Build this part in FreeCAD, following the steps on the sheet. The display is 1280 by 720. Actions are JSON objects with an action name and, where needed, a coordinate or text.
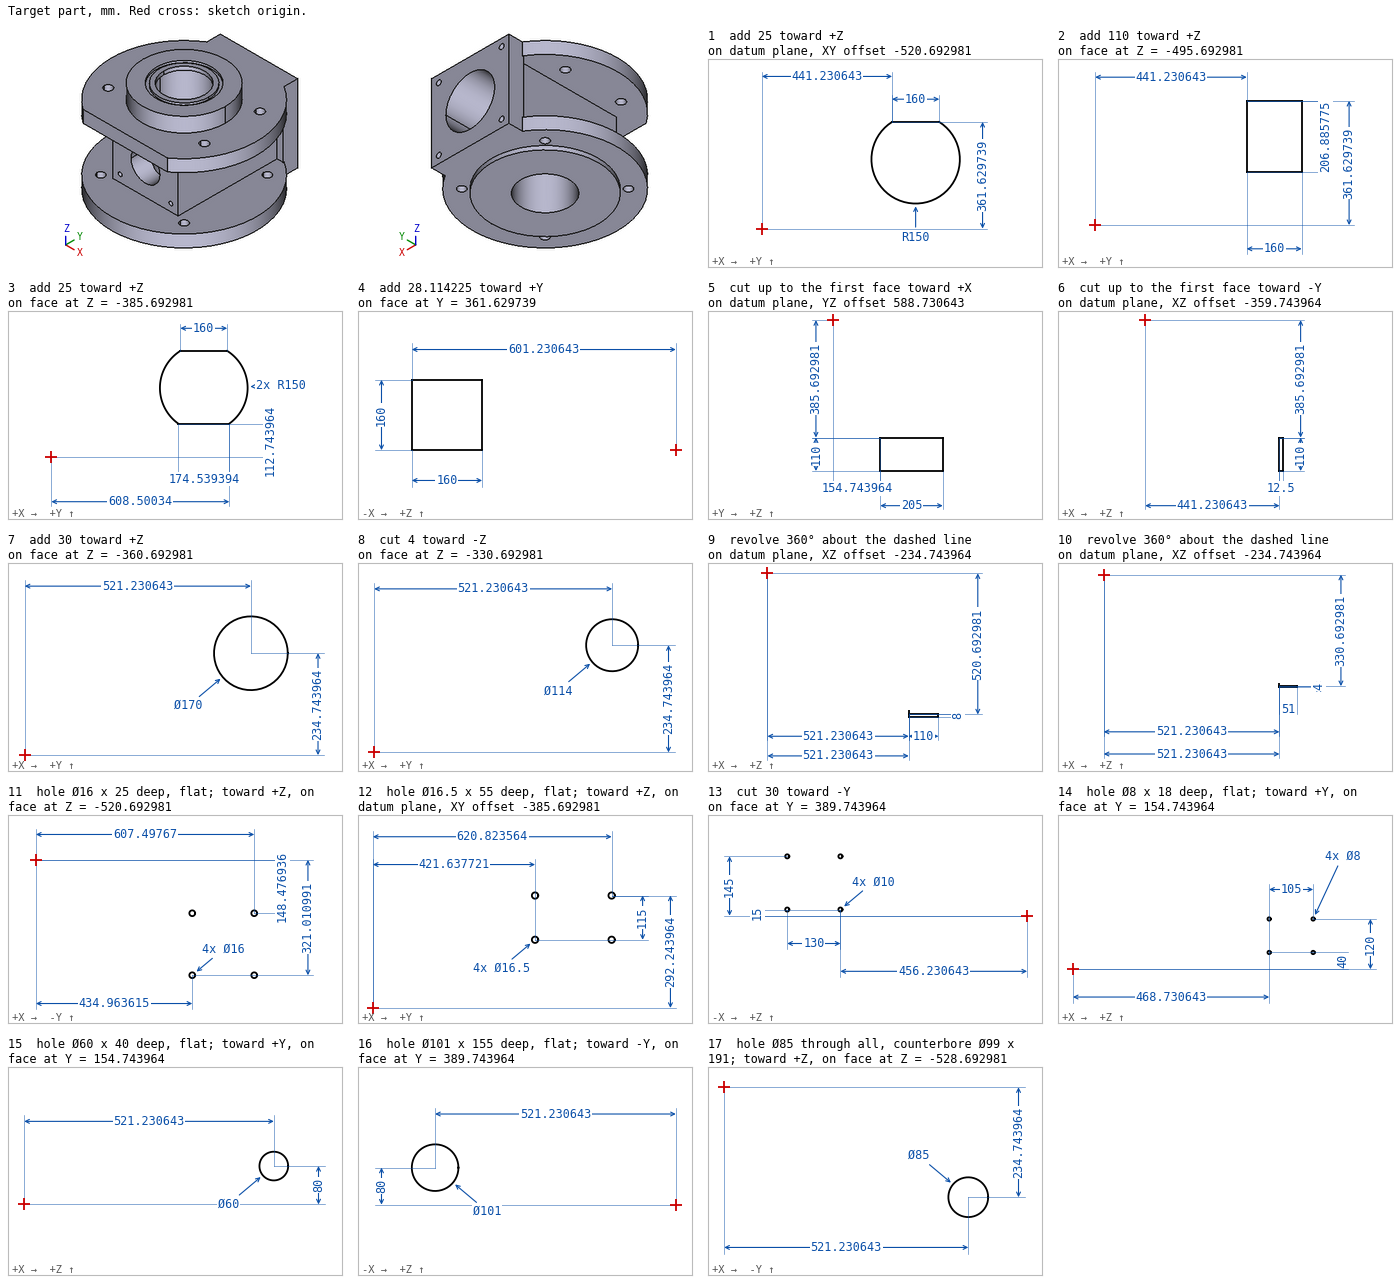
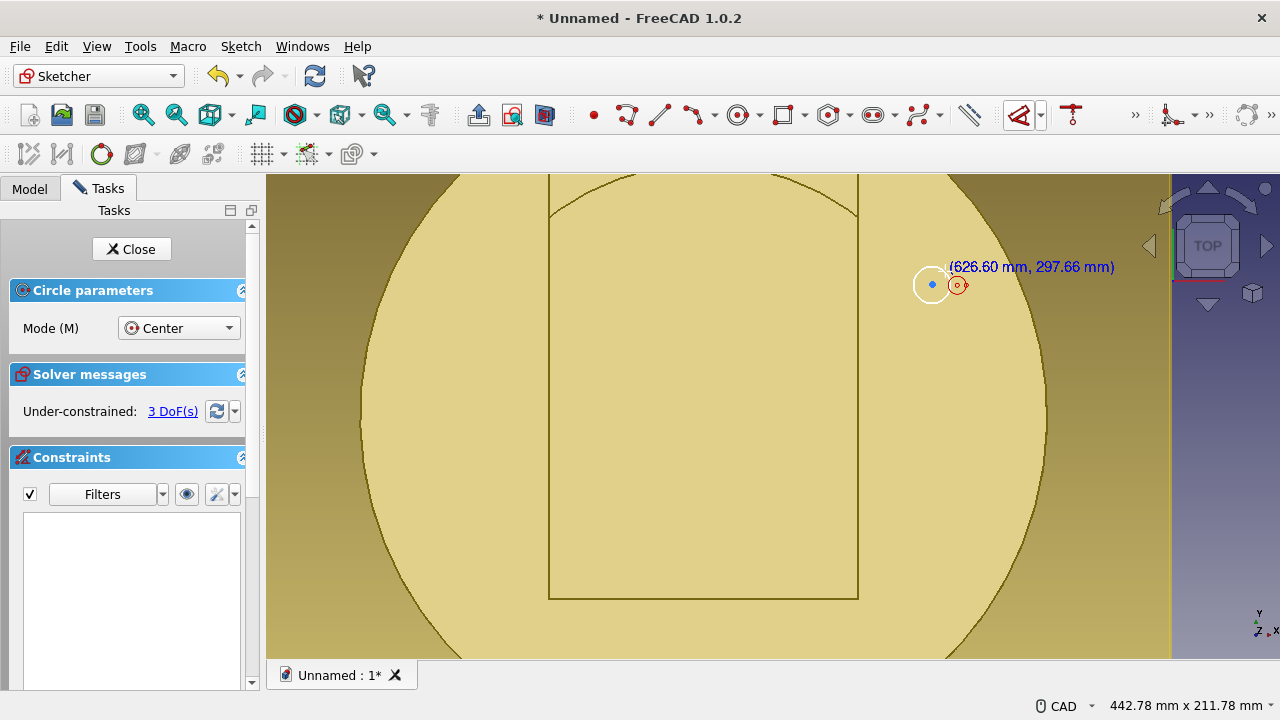
{"action": "left_click", "coordinate": [476, 548]}
{"action": "left_click", "coordinate": [489, 534]}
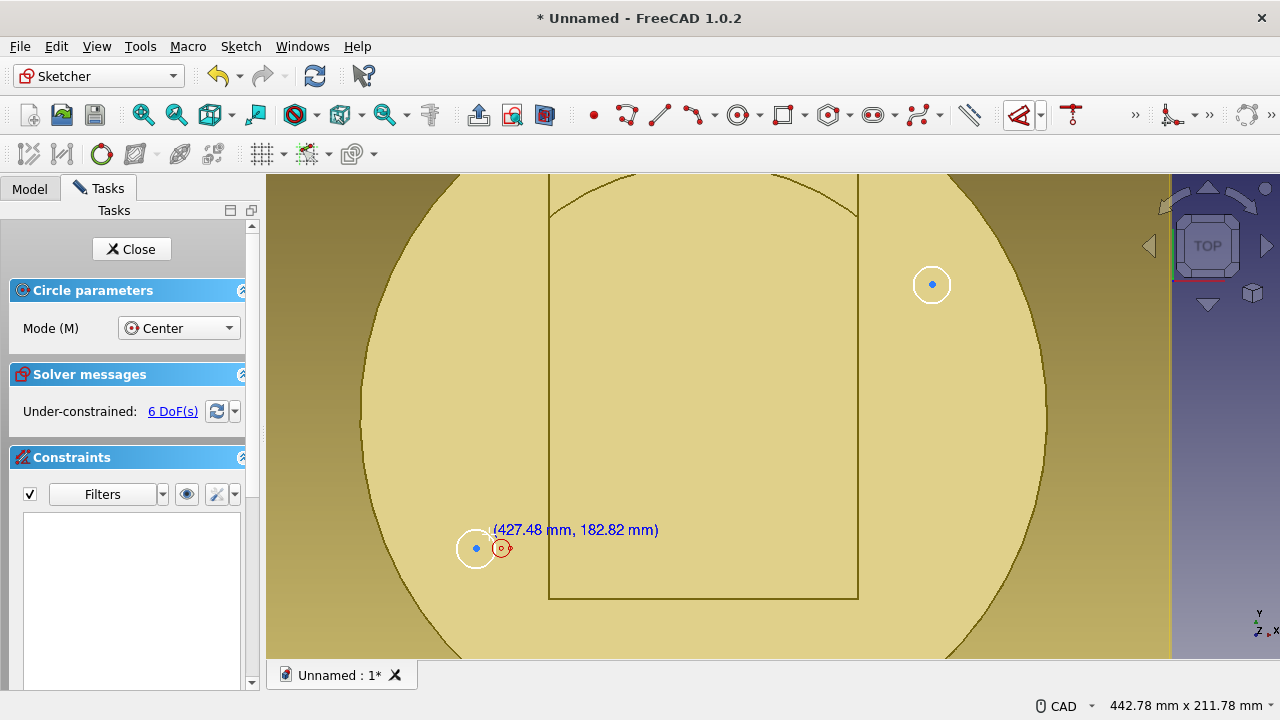
{"action": "left_click", "coordinate": [476, 284]}
{"action": "left_click", "coordinate": [489, 271]}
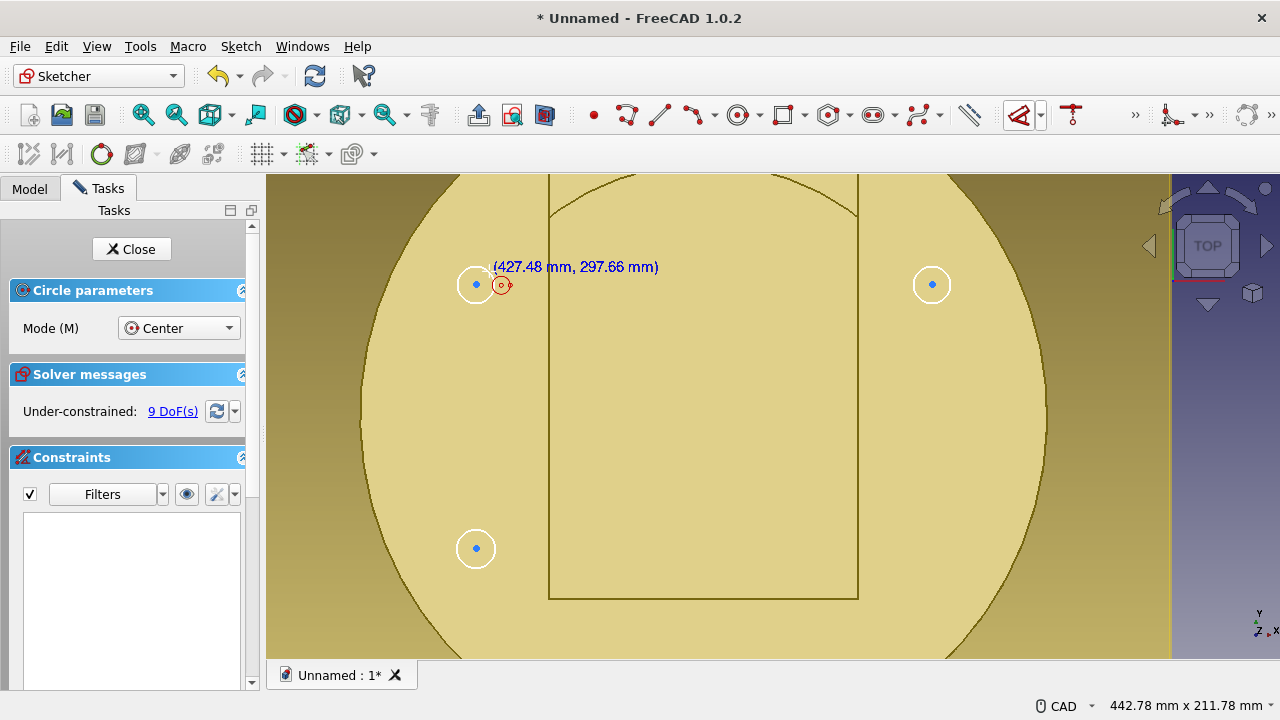
{"action": "left_click", "coordinate": [932, 548]}
{"action": "left_click", "coordinate": [945, 534]}
{"action": "key", "text": "Escape"}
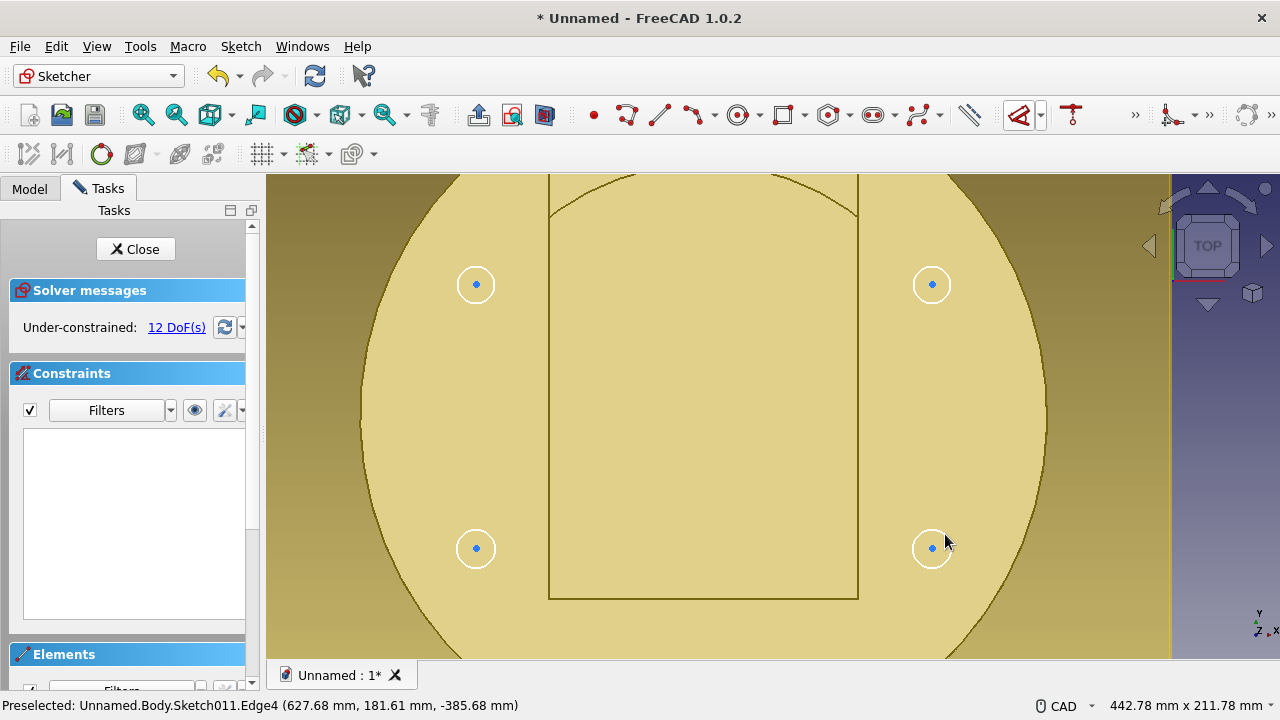
{"action": "left_click", "coordinate": [945, 272]}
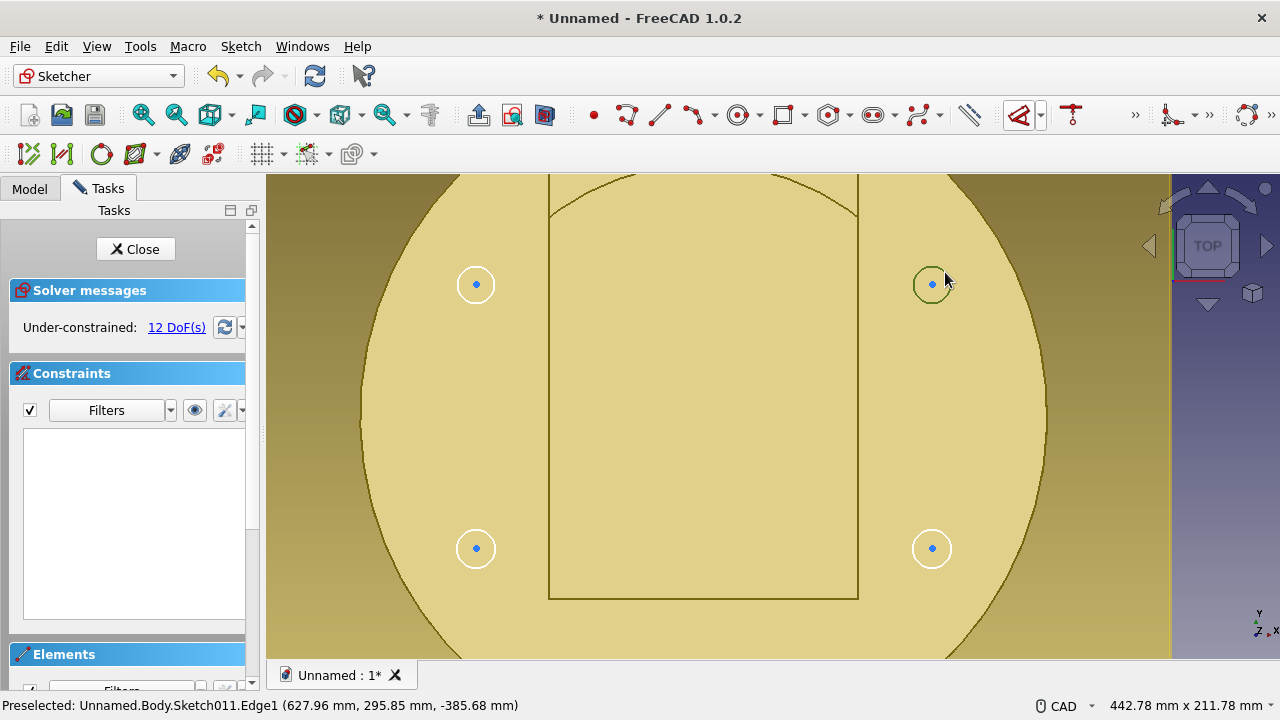
{"action": "left_click", "coordinate": [489, 535]}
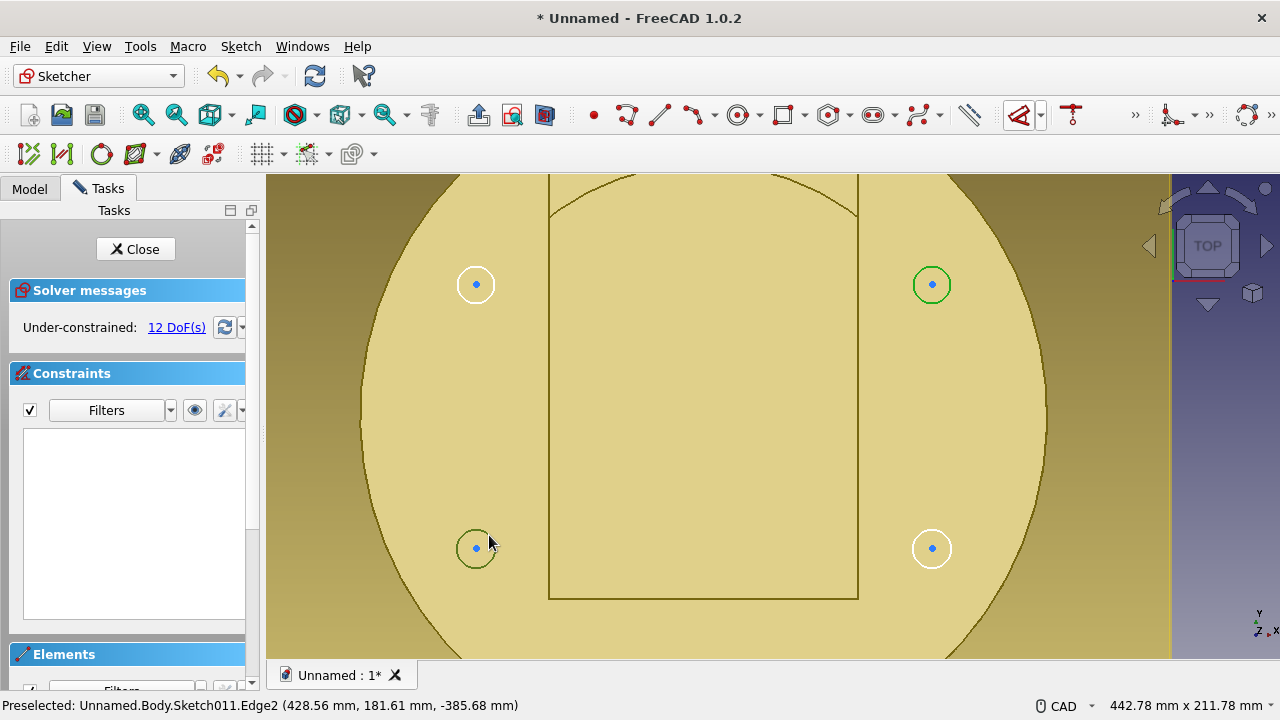
{"action": "left_click", "coordinate": [489, 272]}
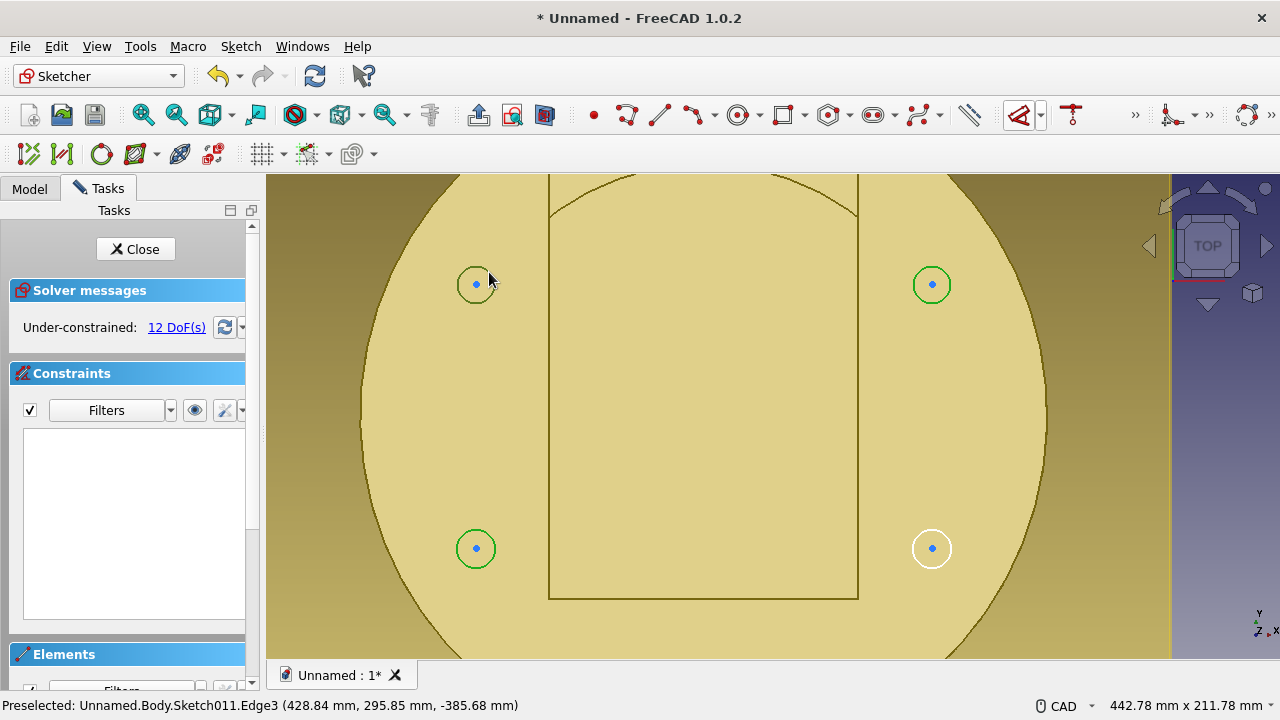
{"action": "left_click", "coordinate": [945, 535]}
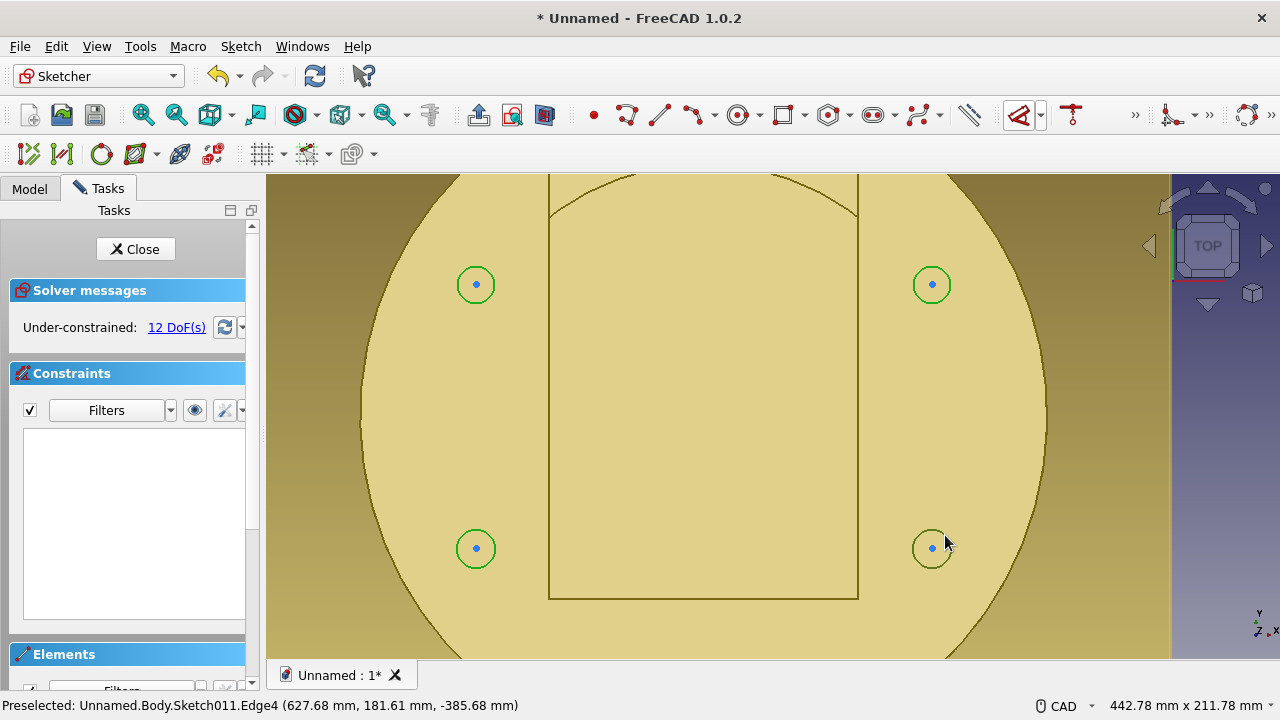
{"action": "key", "text": "e"}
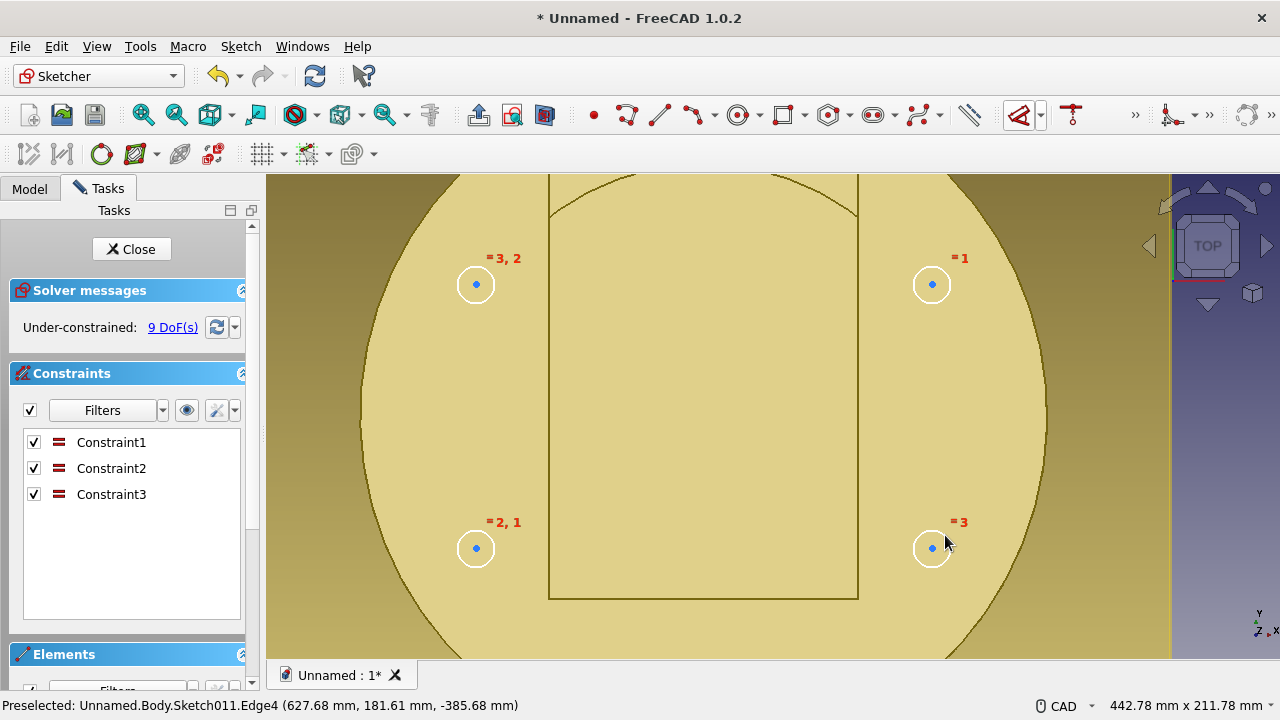
{"action": "left_click", "coordinate": [476, 549]}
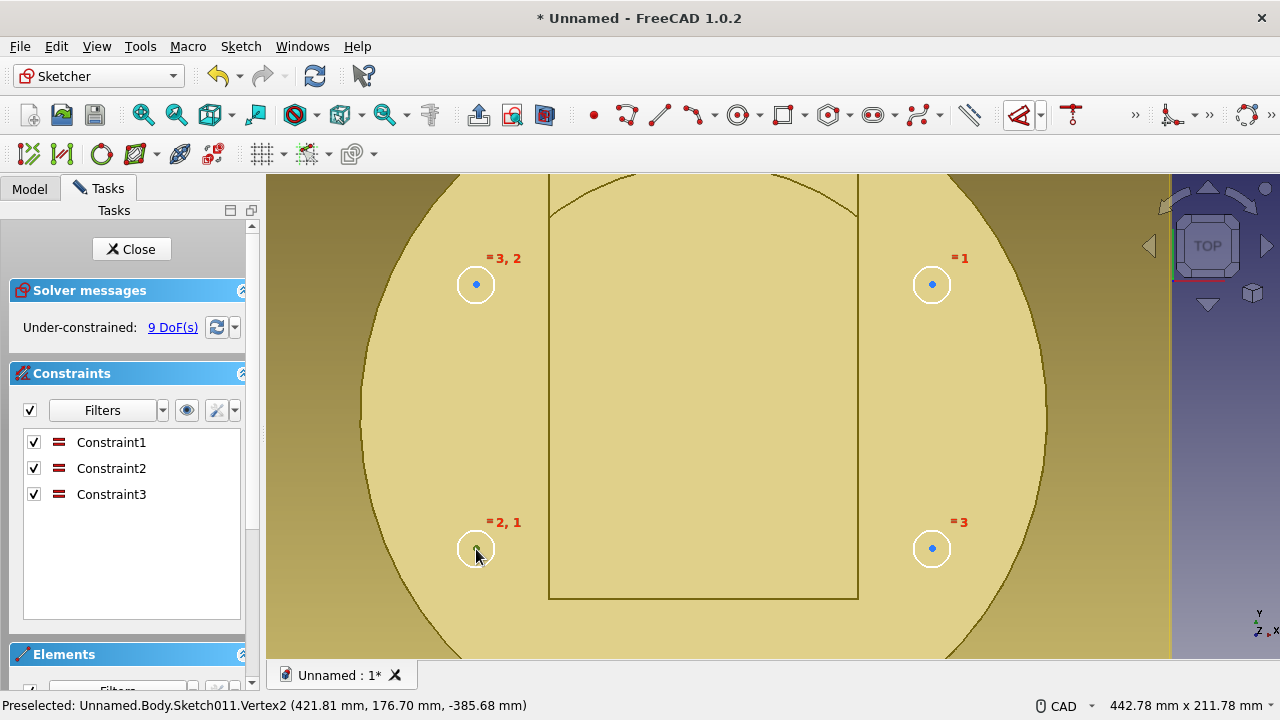
{"action": "left_click", "coordinate": [476, 285]}